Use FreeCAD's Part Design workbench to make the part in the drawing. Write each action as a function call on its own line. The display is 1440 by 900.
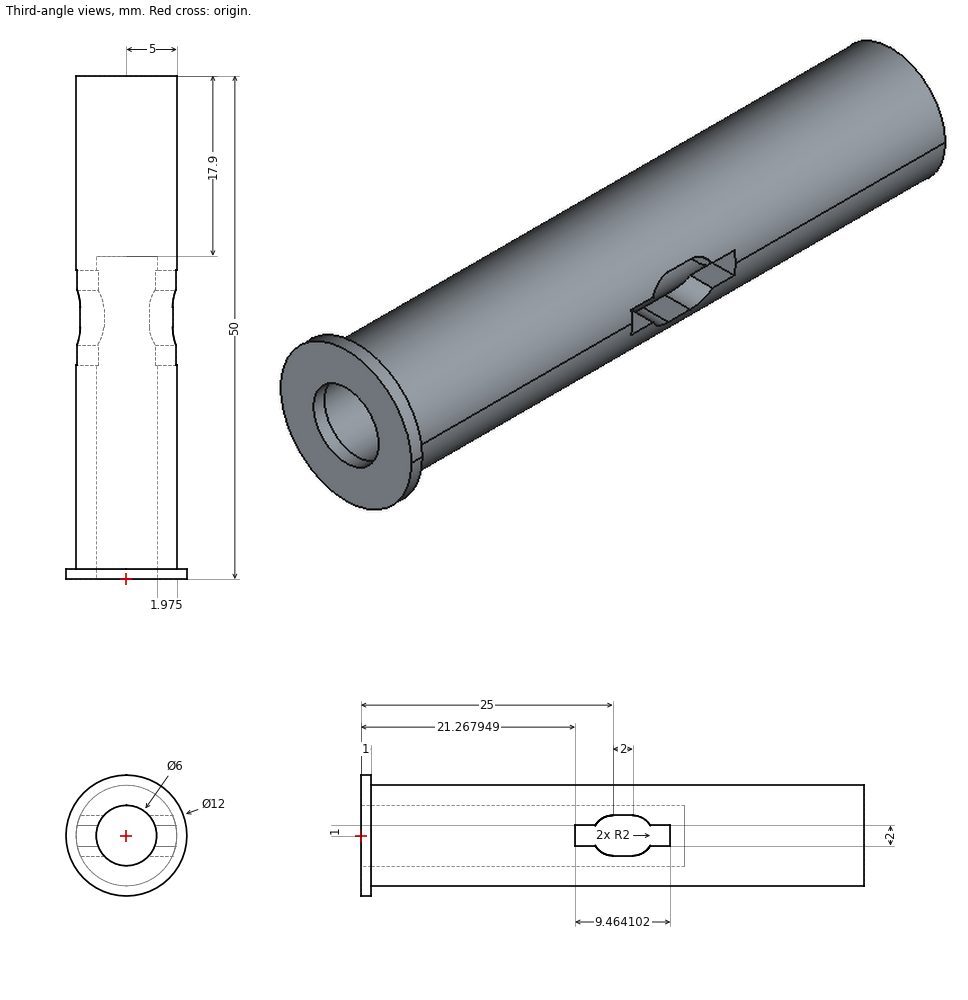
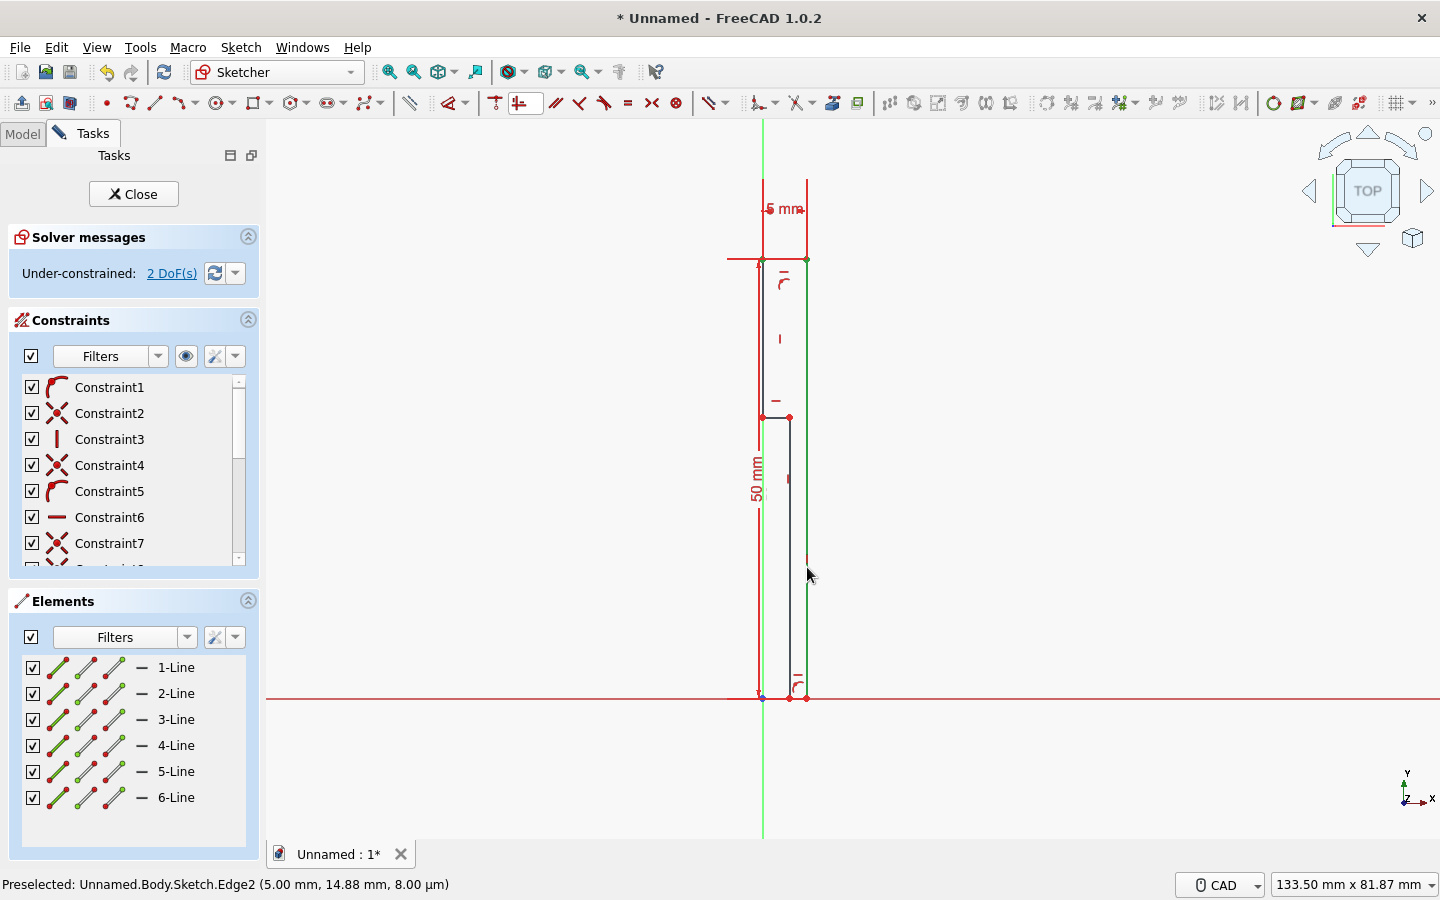
click(763, 307)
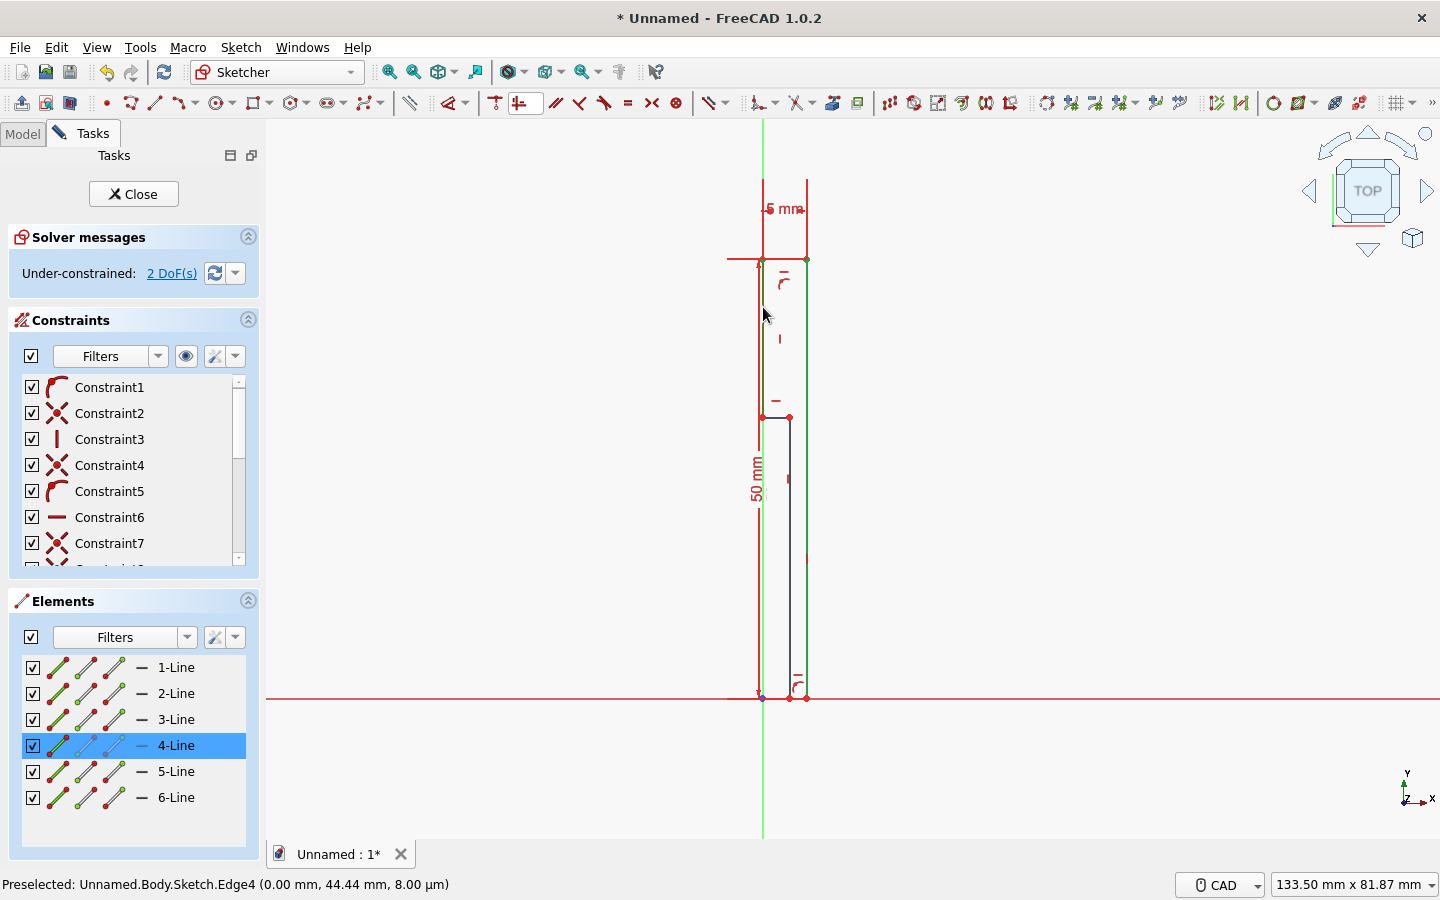
key(i)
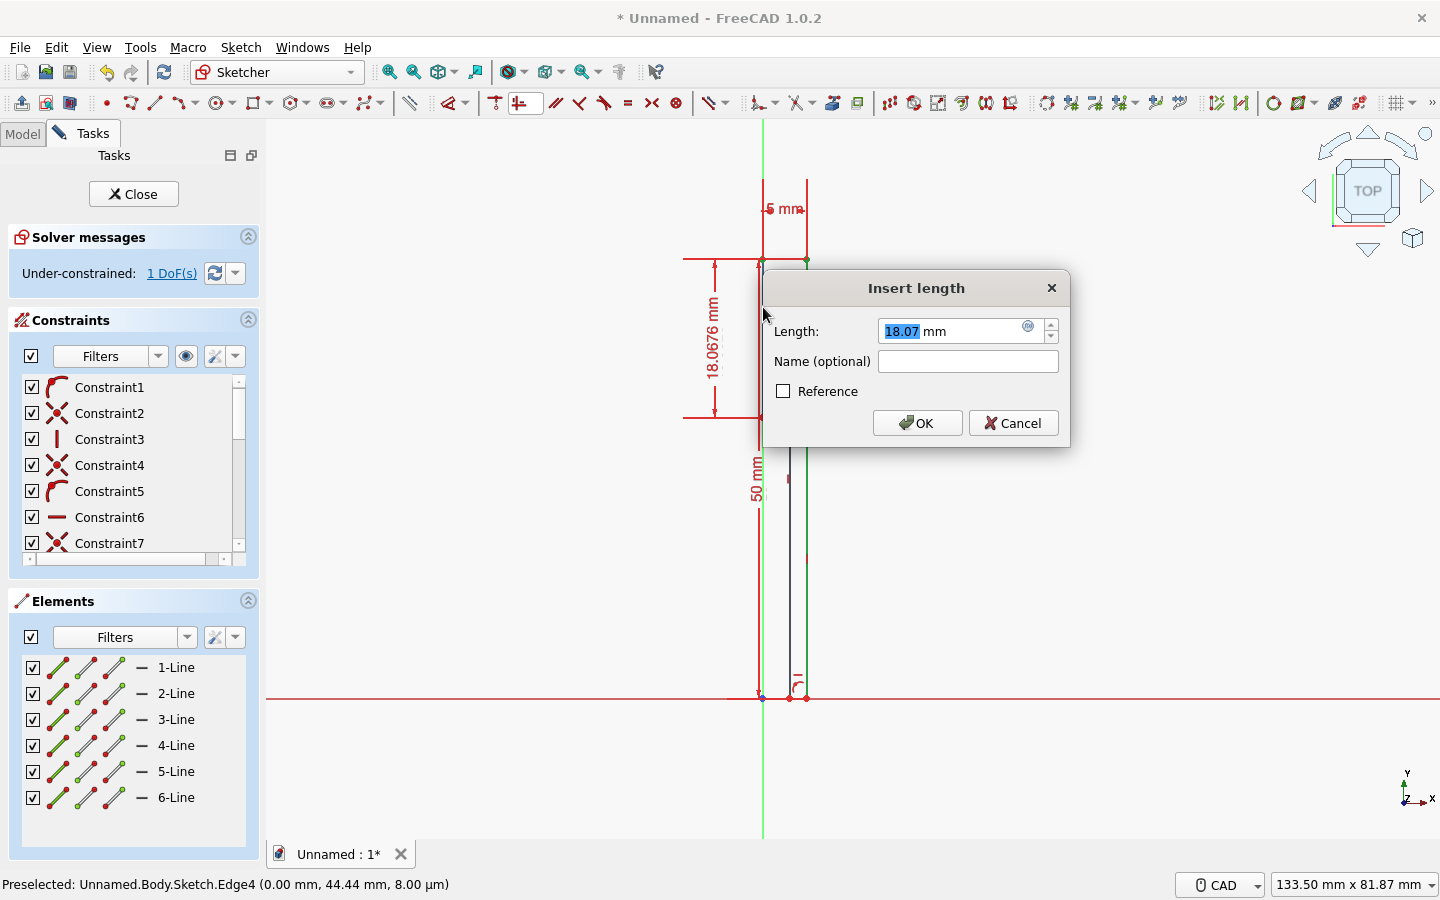
text(17.9)
key(Return)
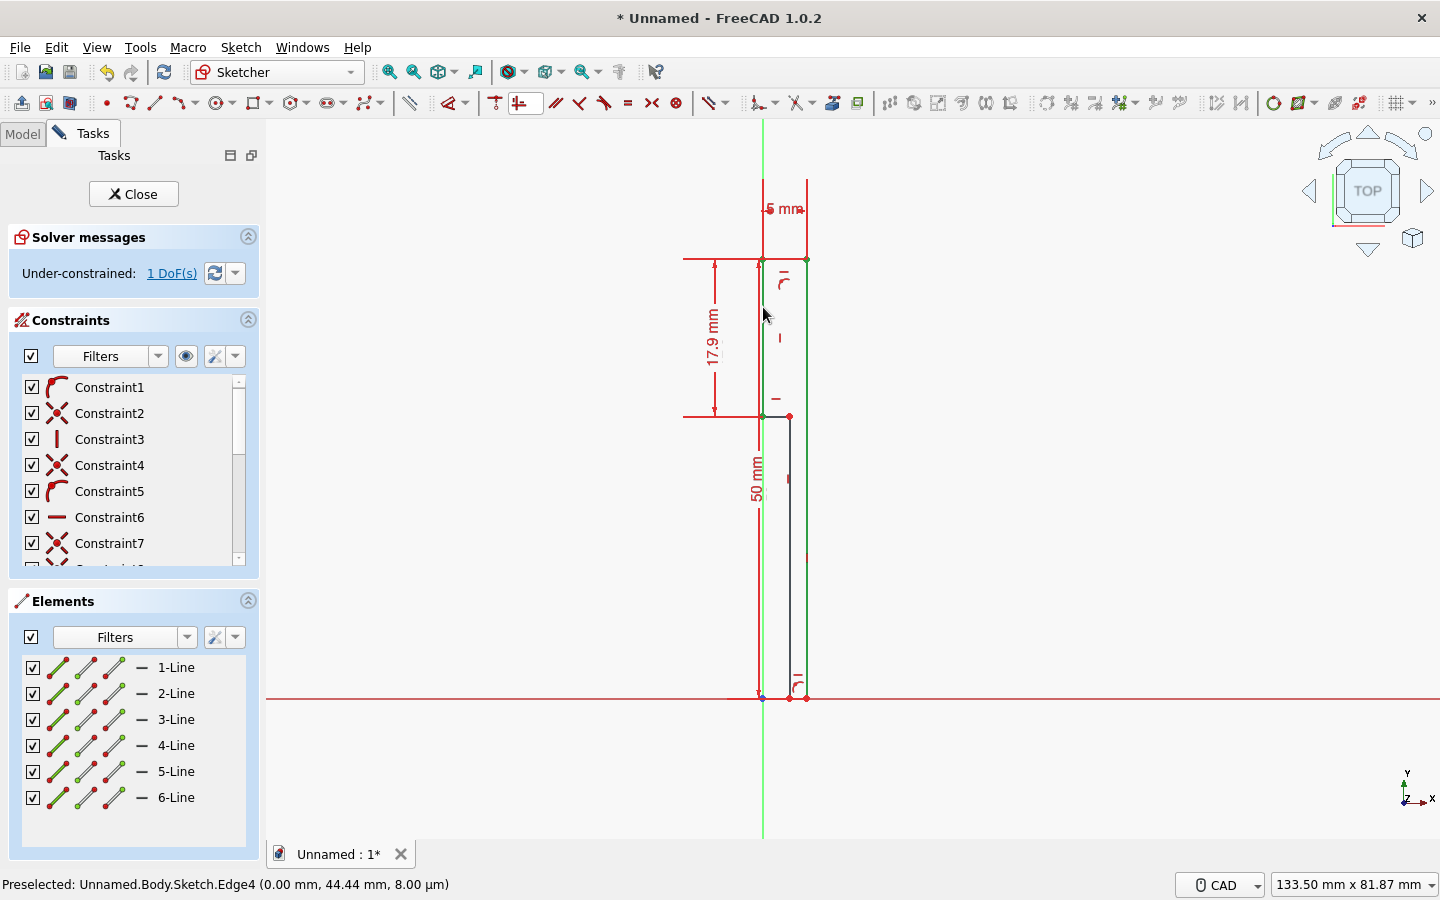
scroll(798, 699, up, 5)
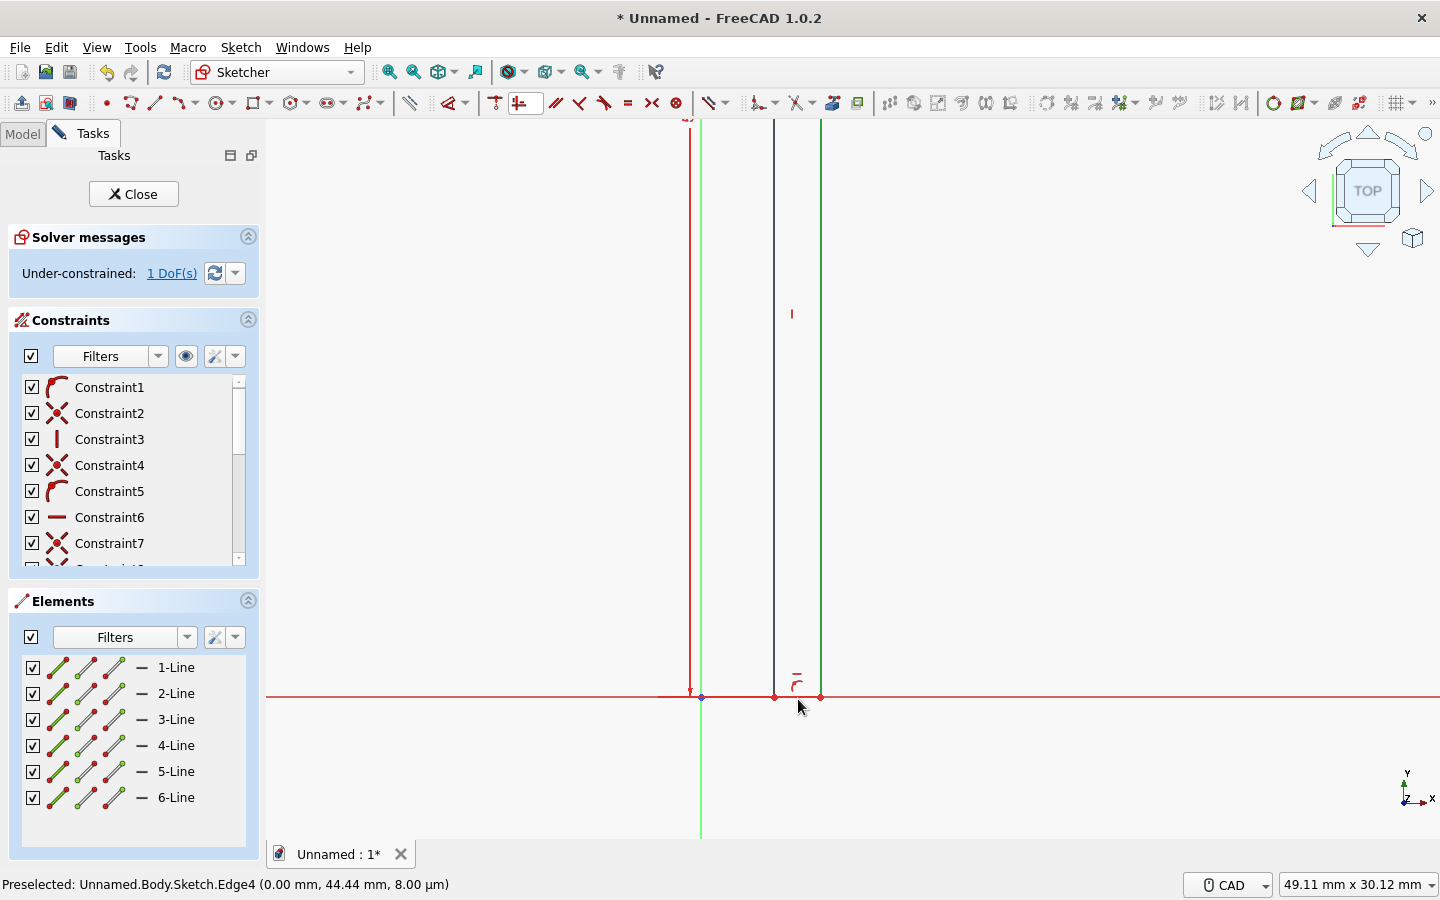
click(797, 697)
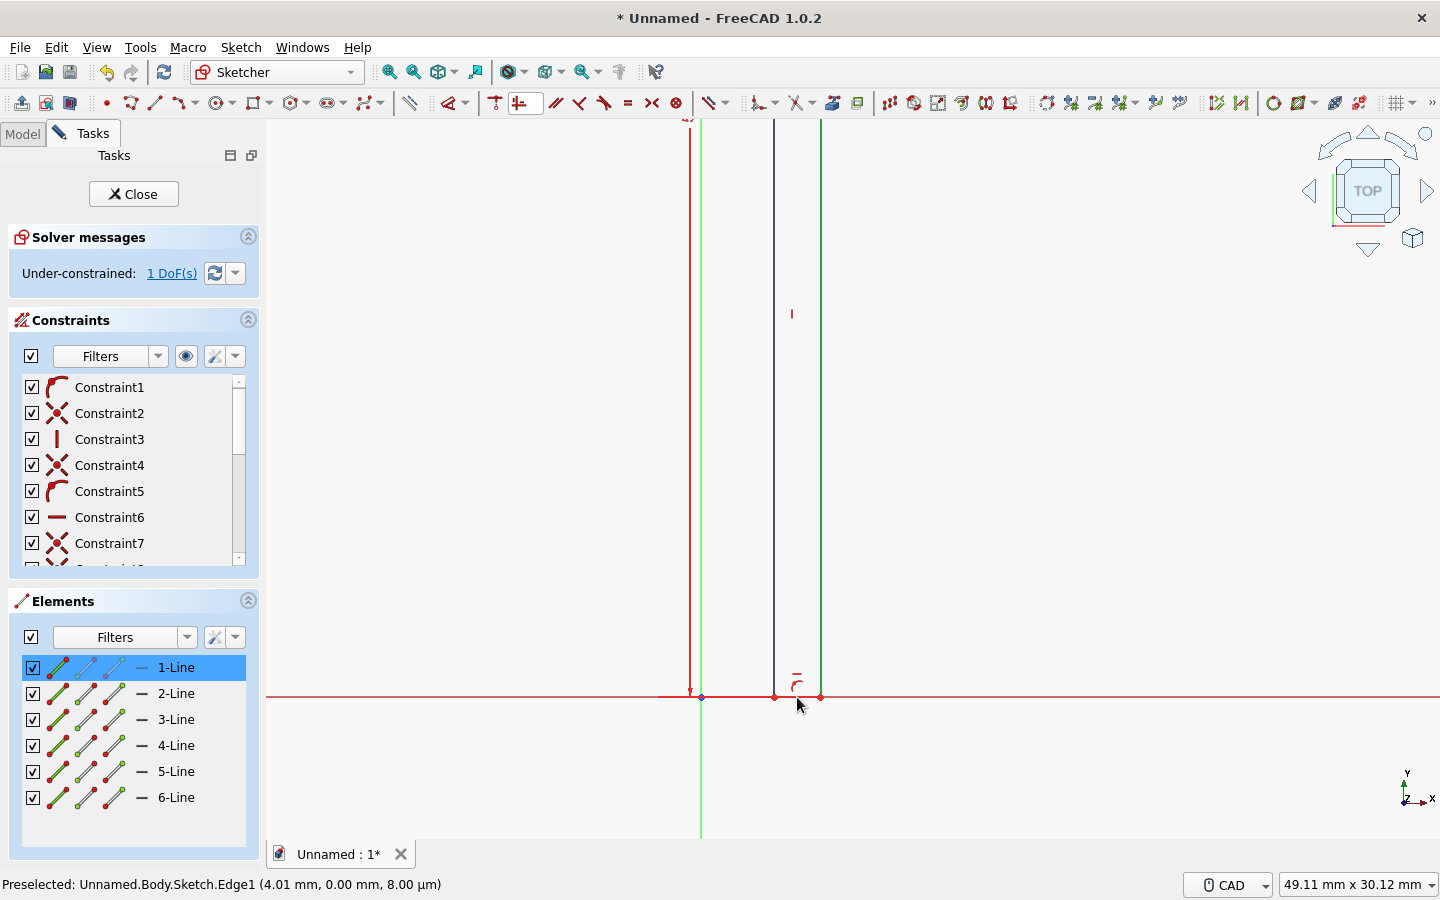
click(468, 104)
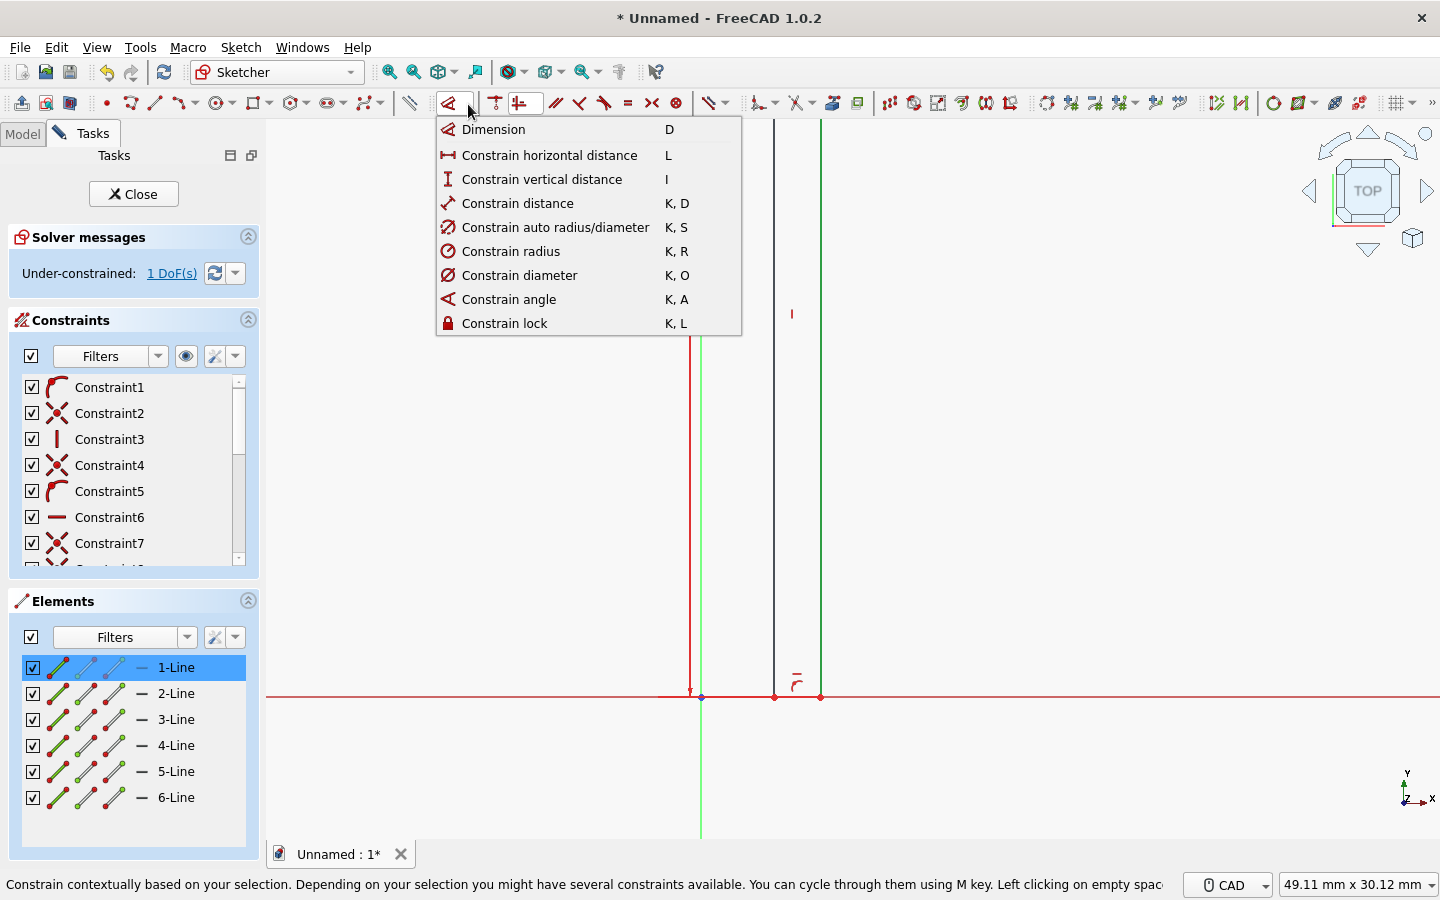
click(589, 155)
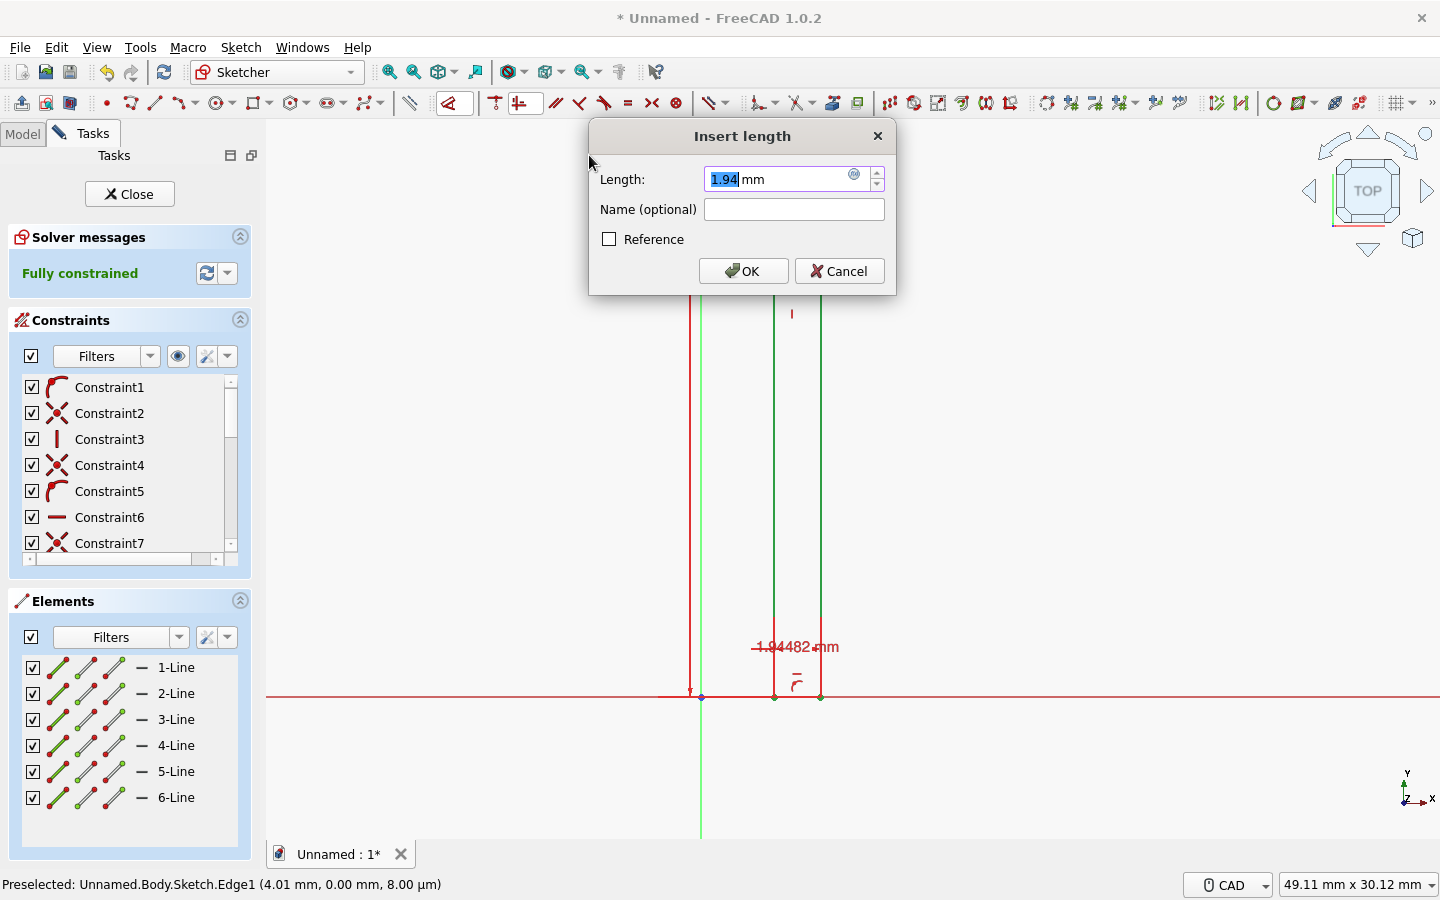
text(1.975)
key(Return)